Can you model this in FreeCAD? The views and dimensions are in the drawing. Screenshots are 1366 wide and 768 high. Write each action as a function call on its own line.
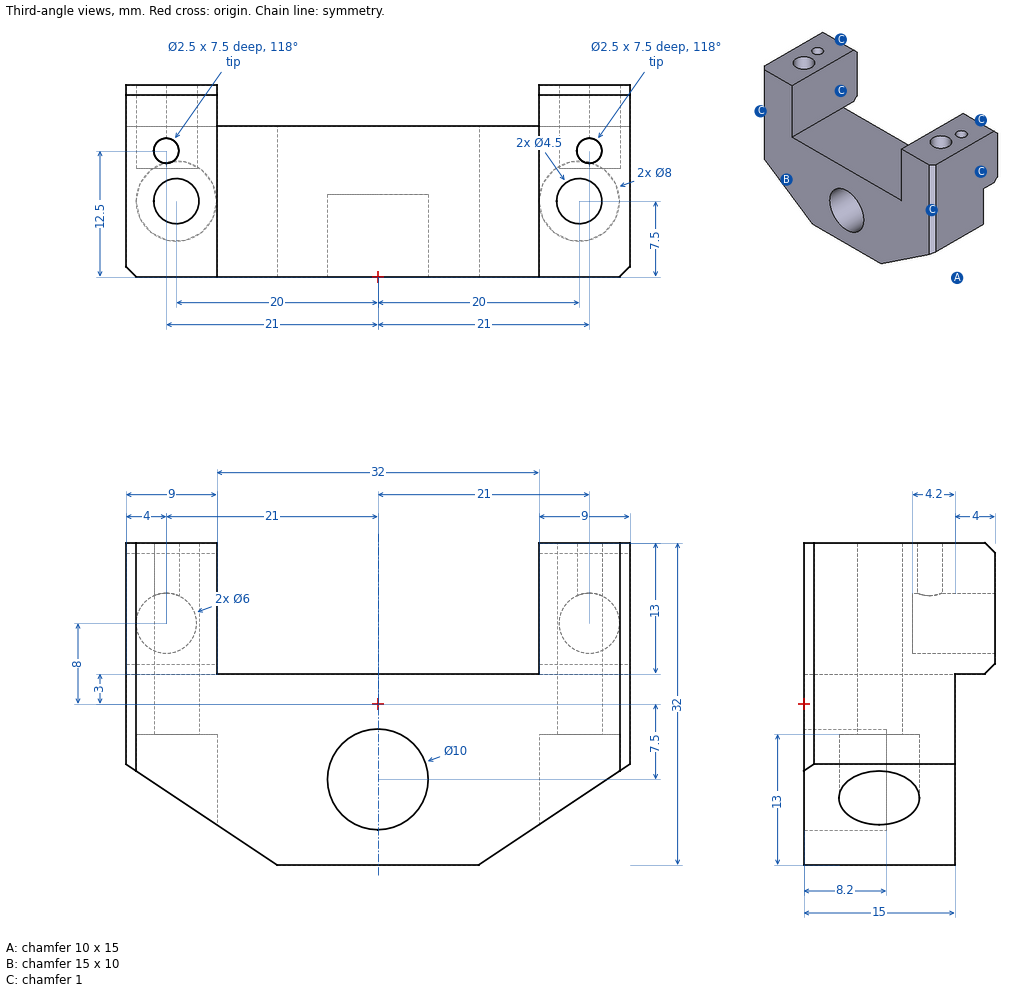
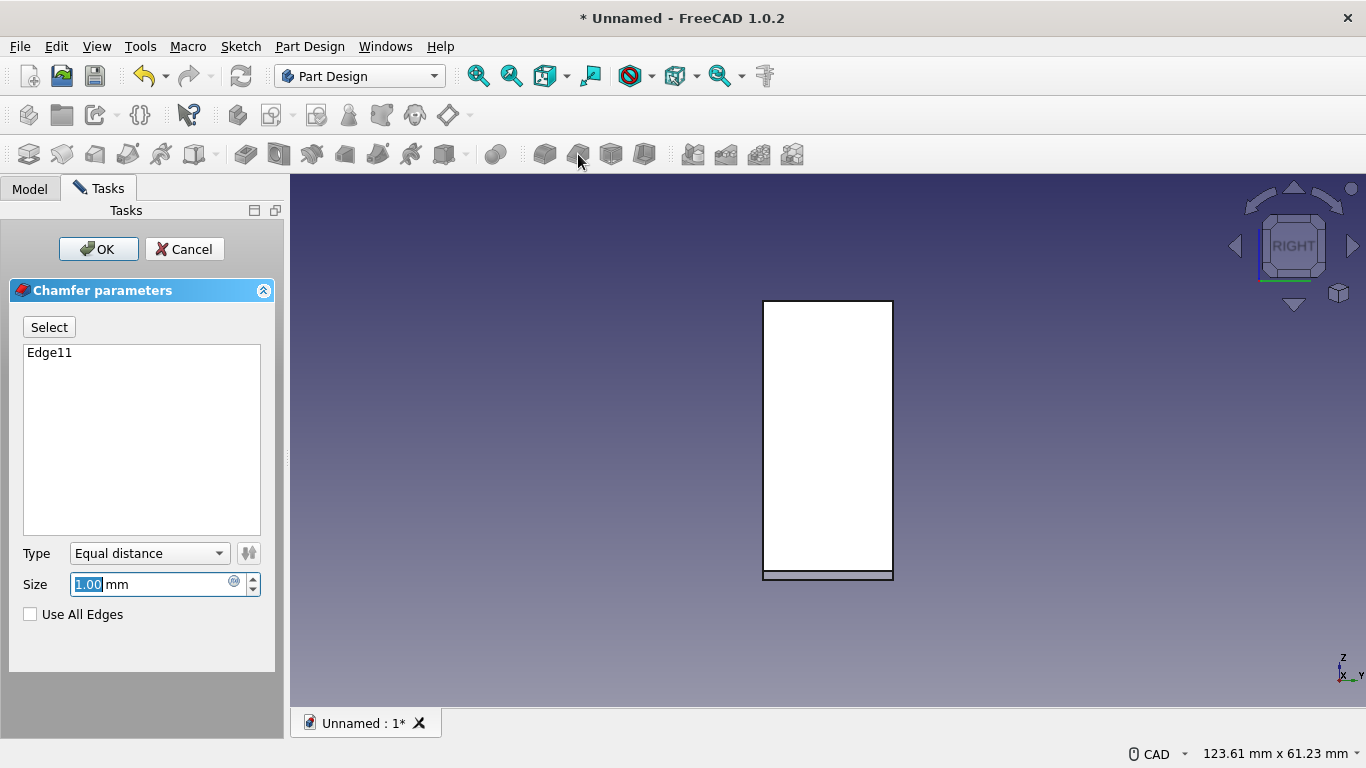
text(10)
key(Tab)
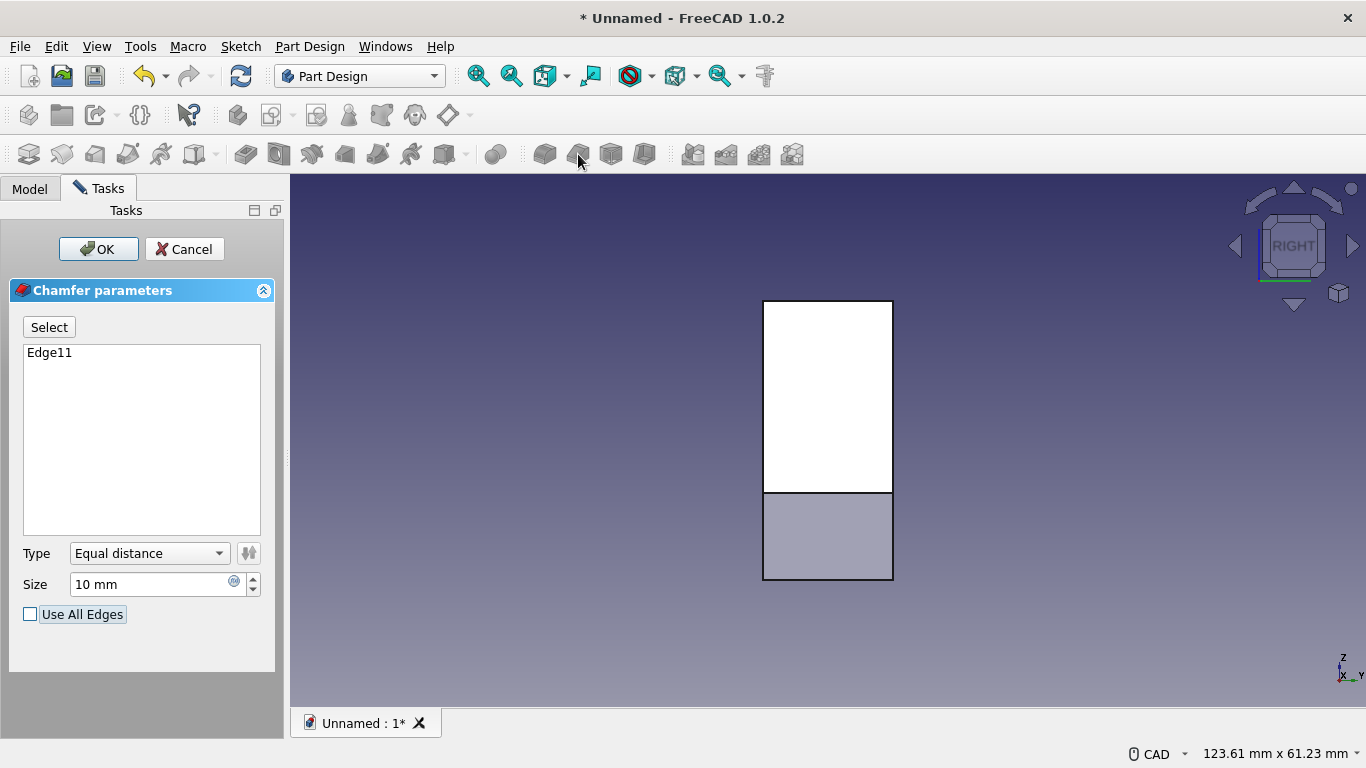
click(150, 554)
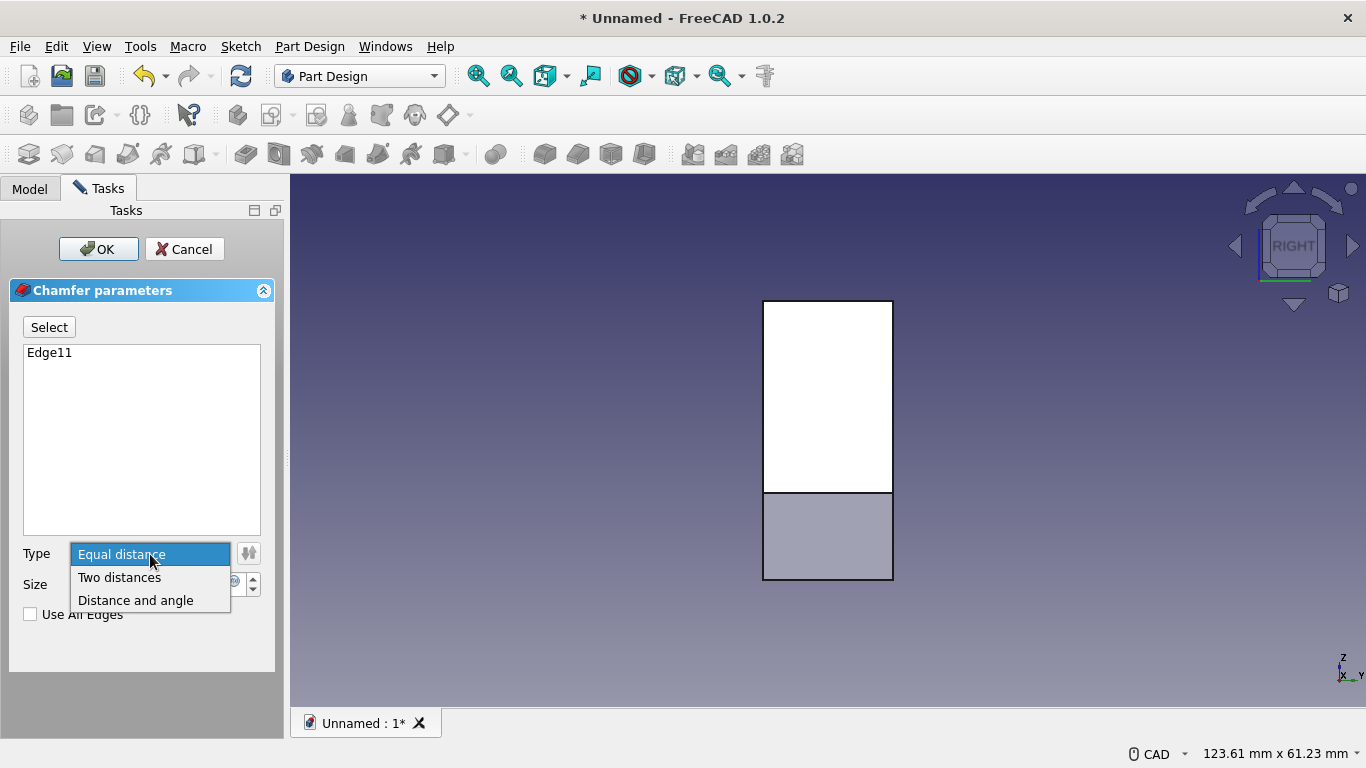
click(148, 578)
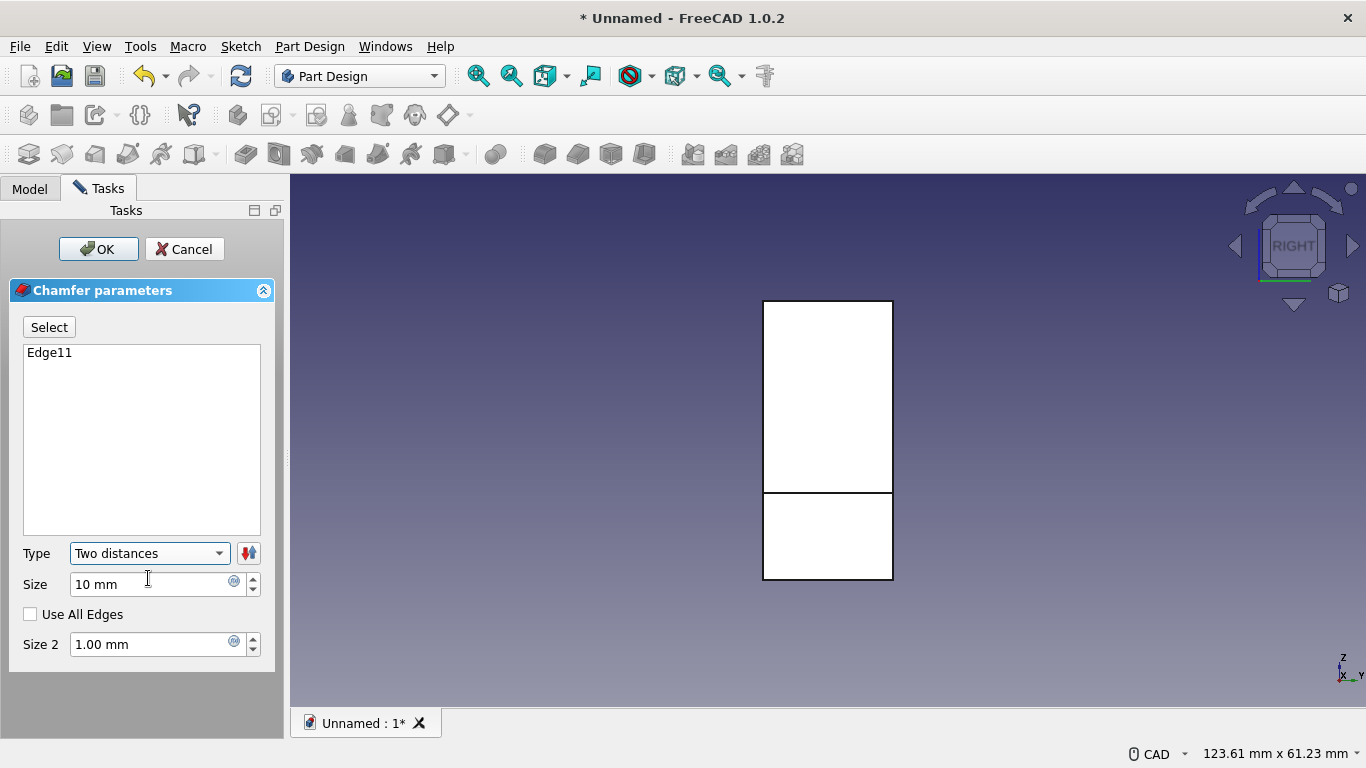
triple_click(158, 644)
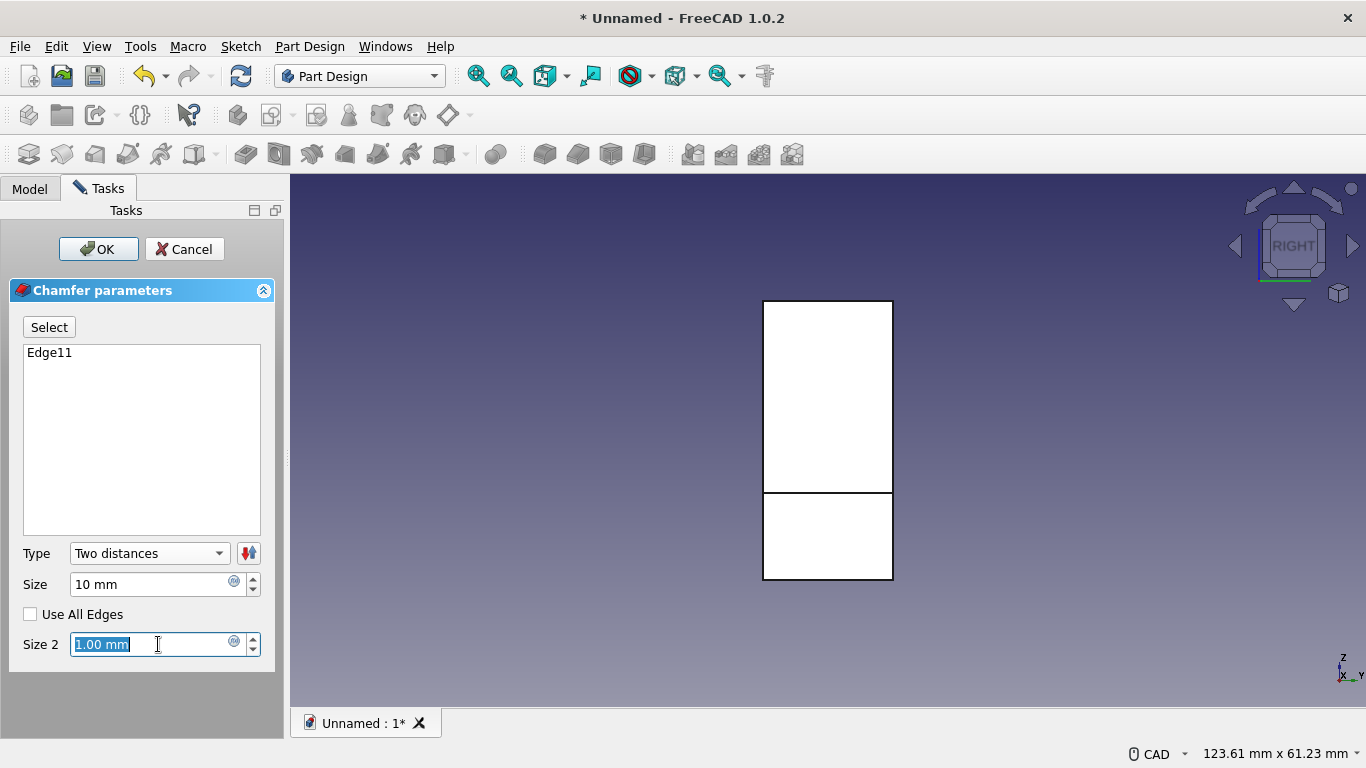
text(15)
key(Tab)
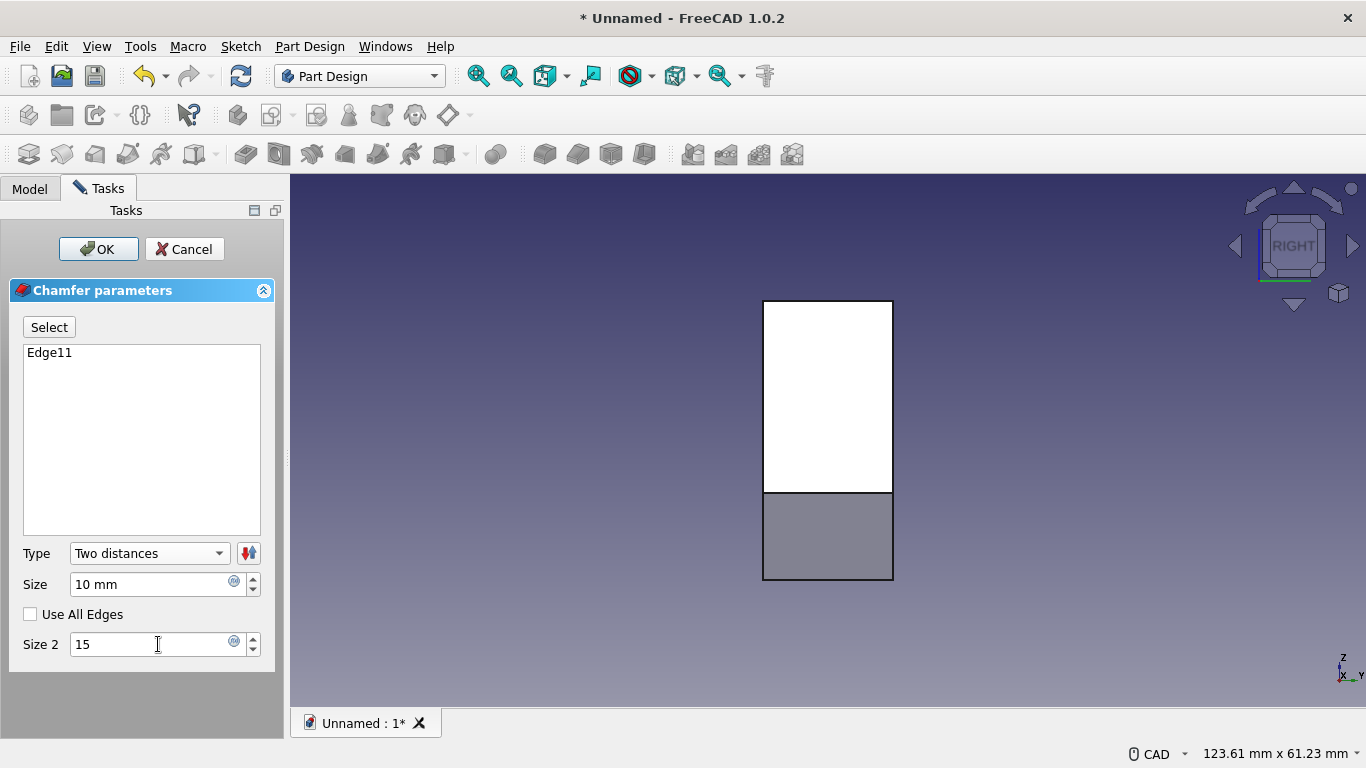
click(99, 249)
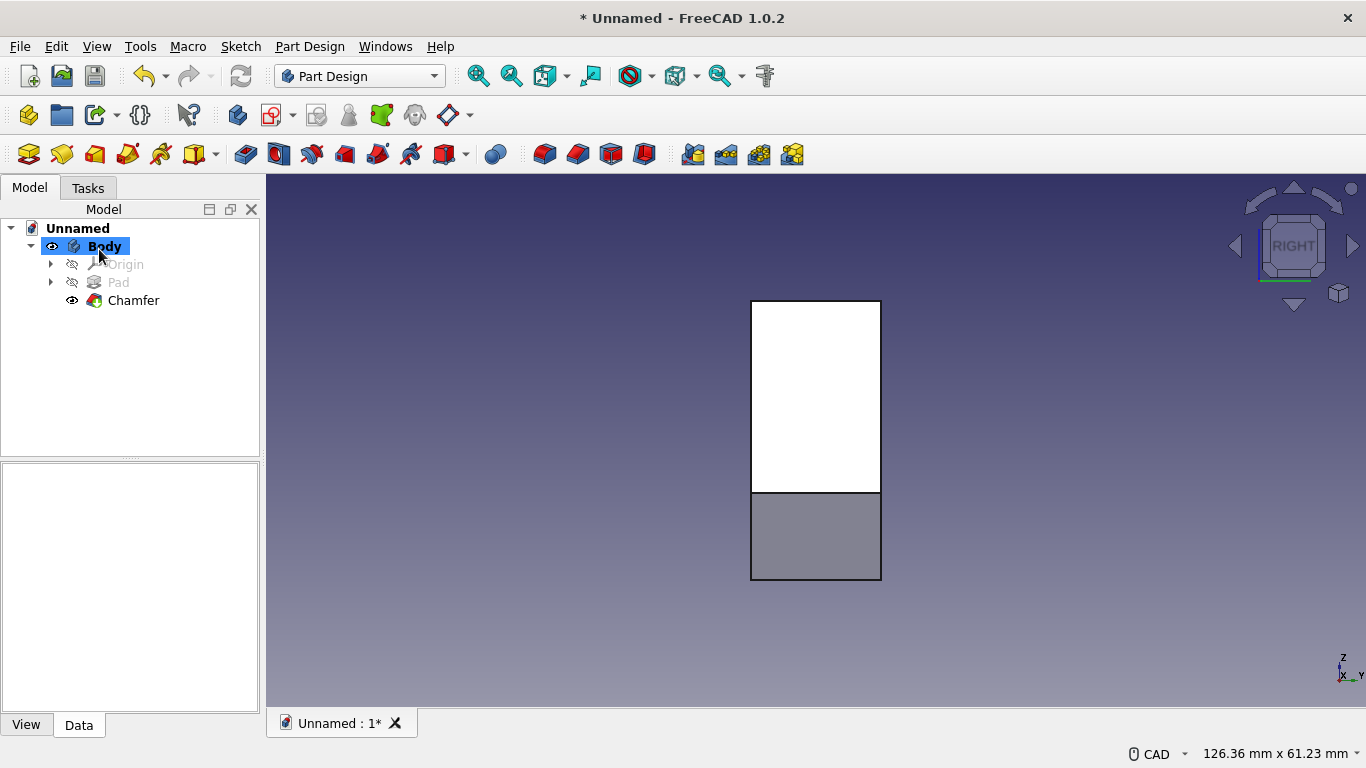
key(0)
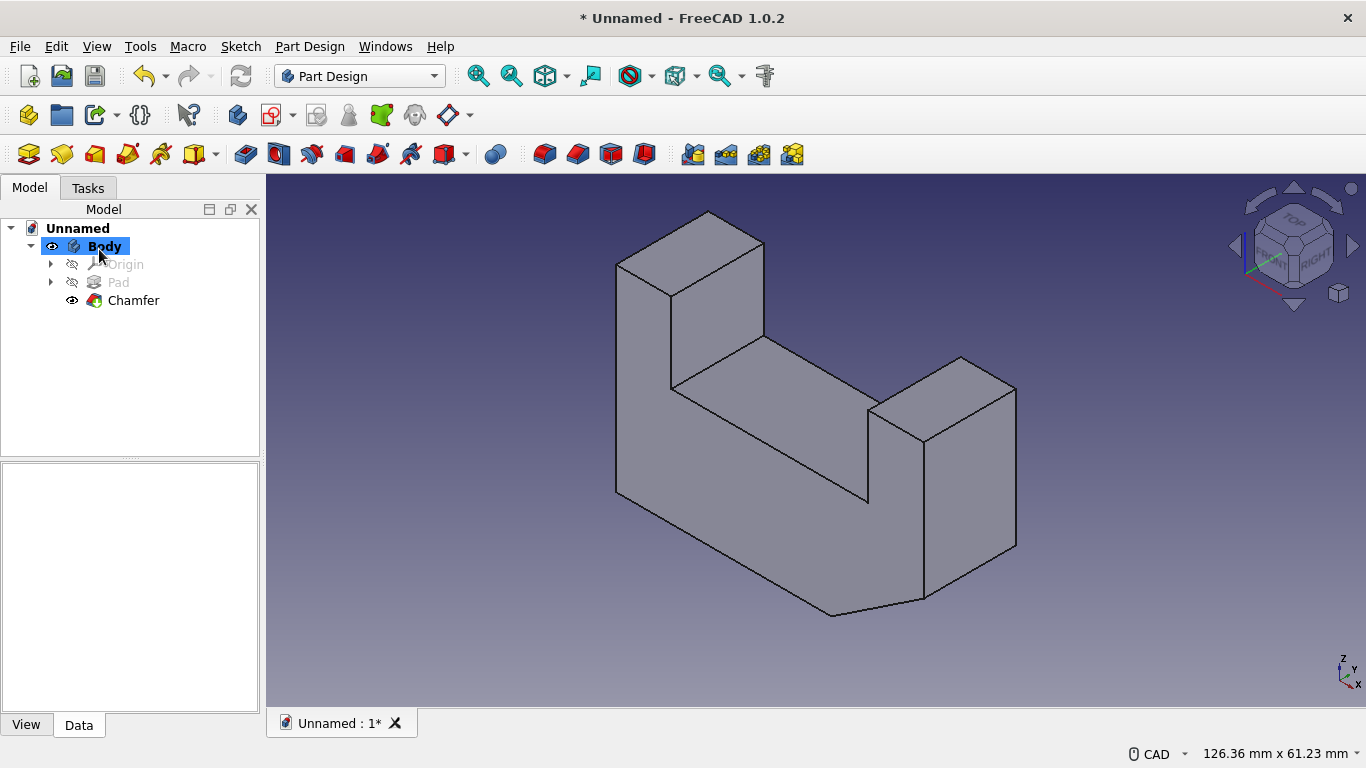
key(2)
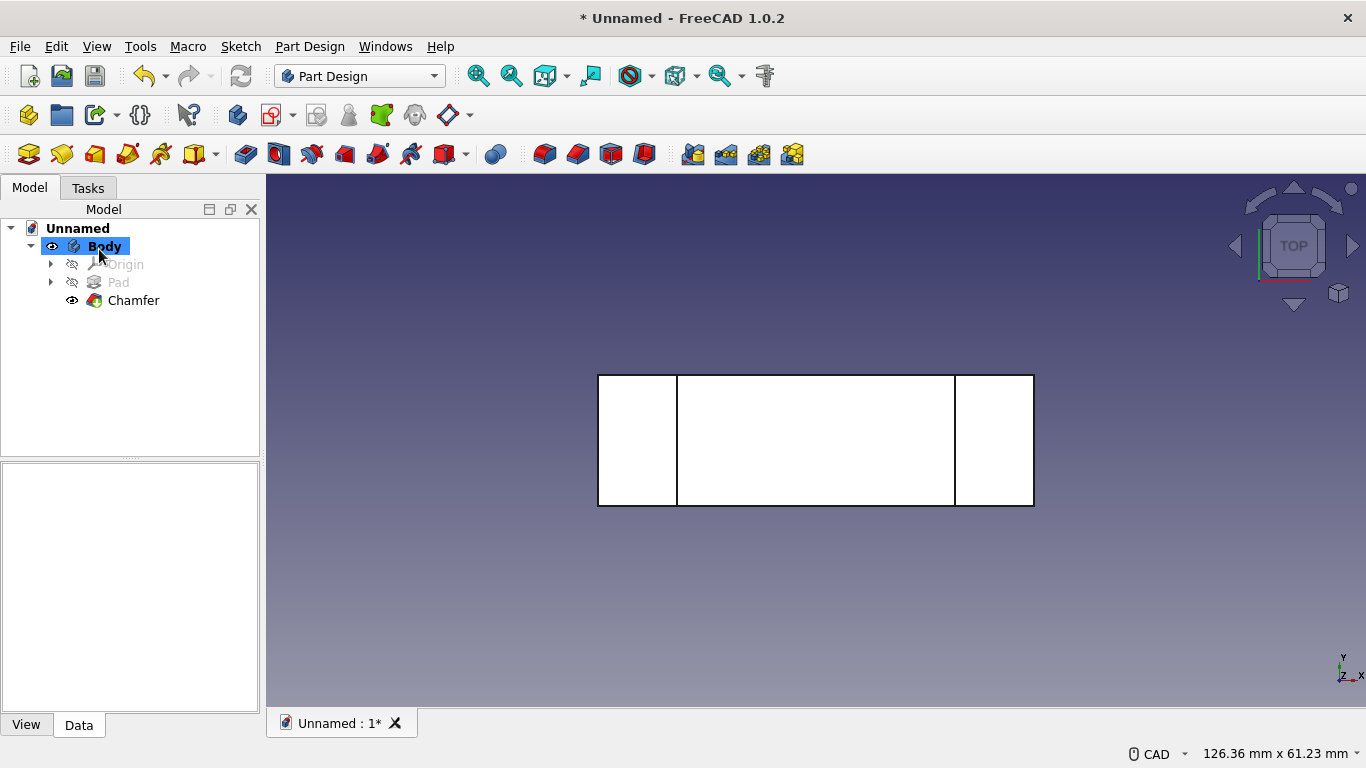
key(v)
key(f)